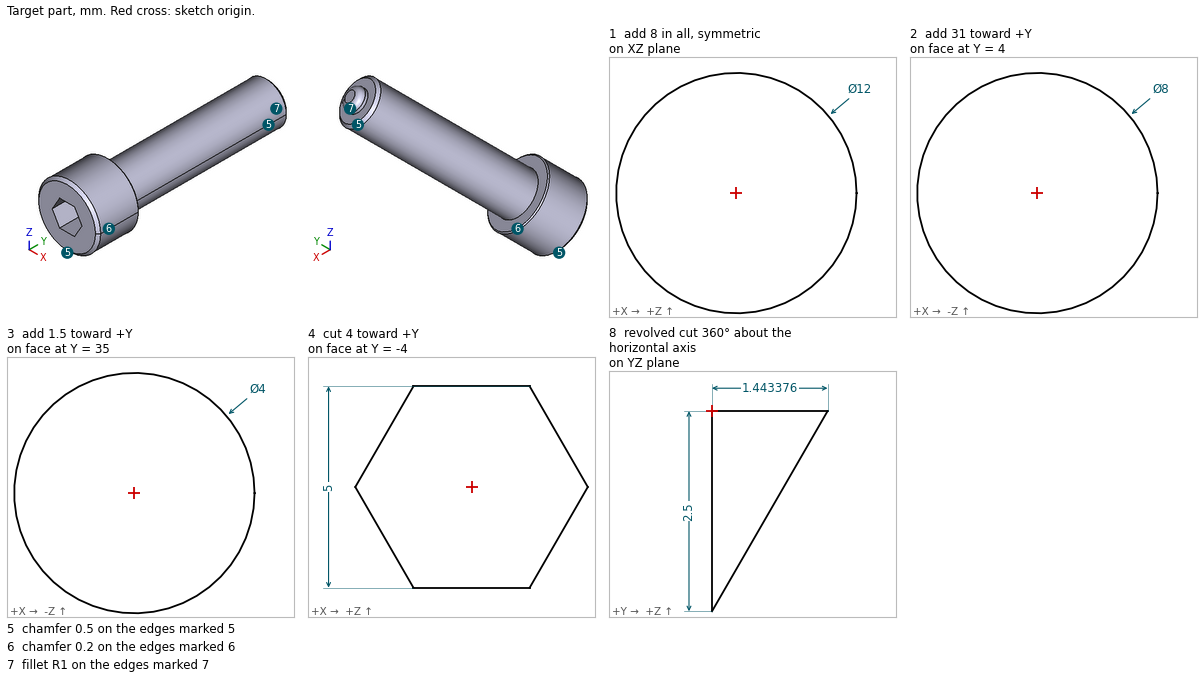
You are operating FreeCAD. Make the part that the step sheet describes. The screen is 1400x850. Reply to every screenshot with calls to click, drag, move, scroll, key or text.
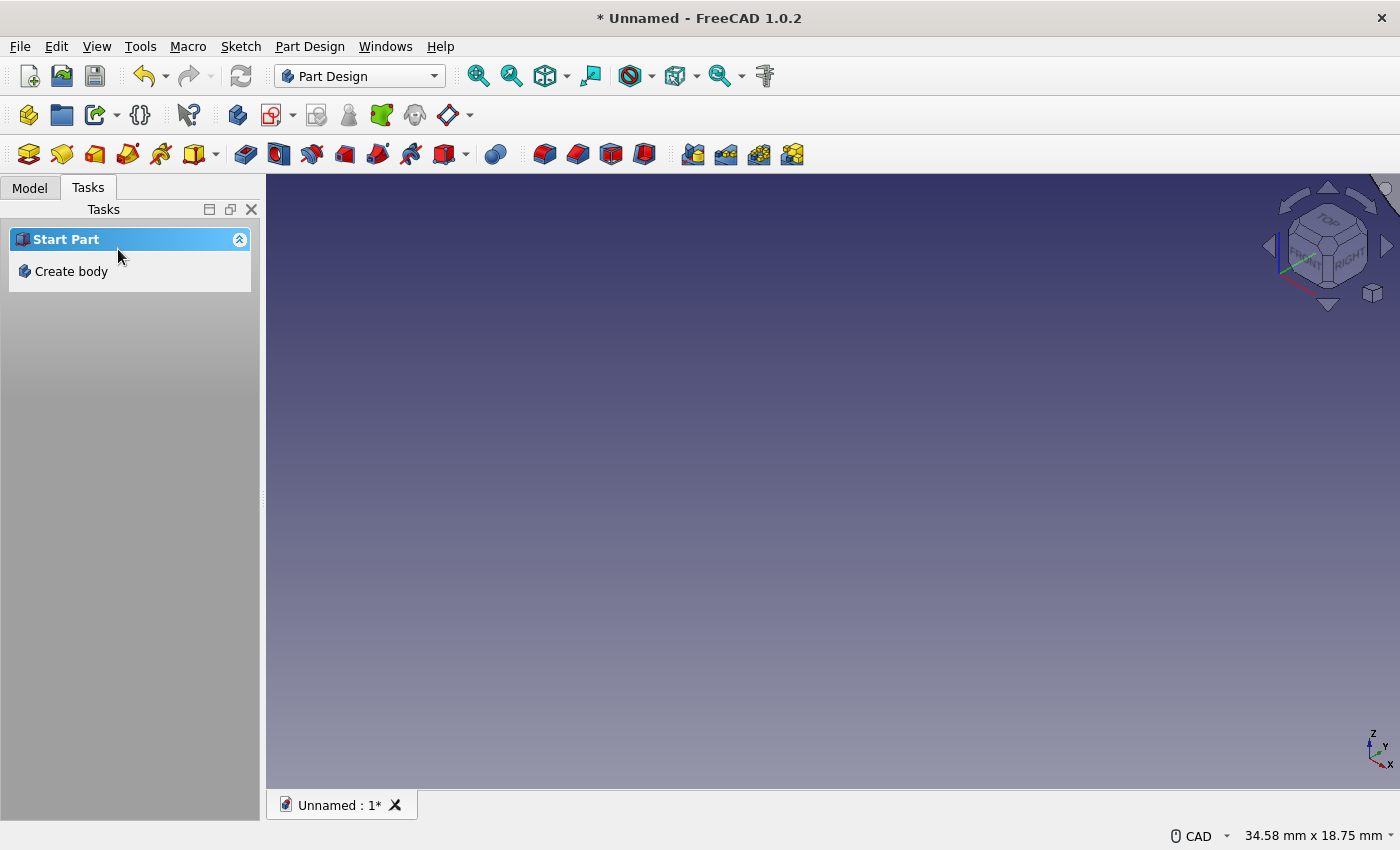
click(479, 76)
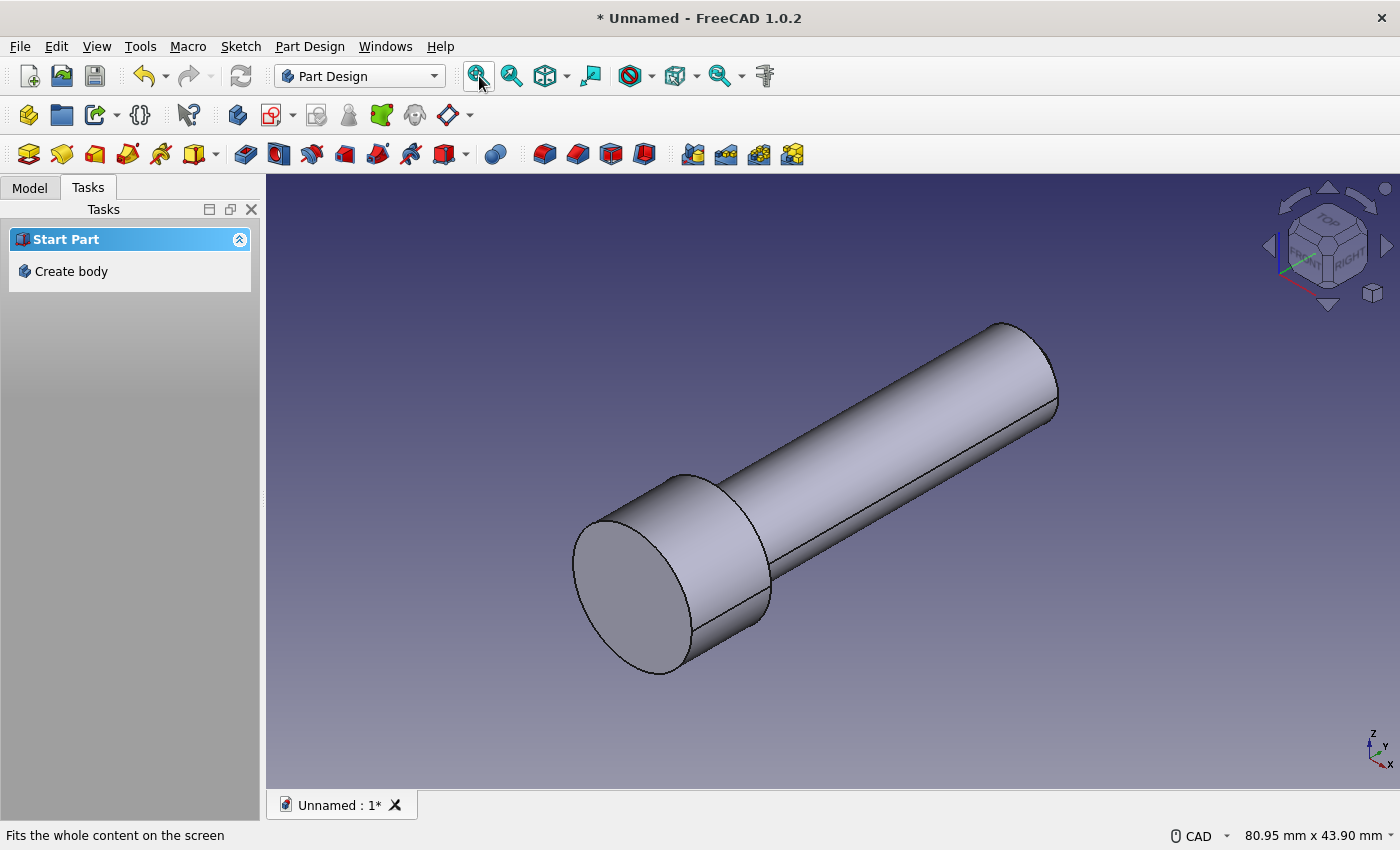
click(632, 596)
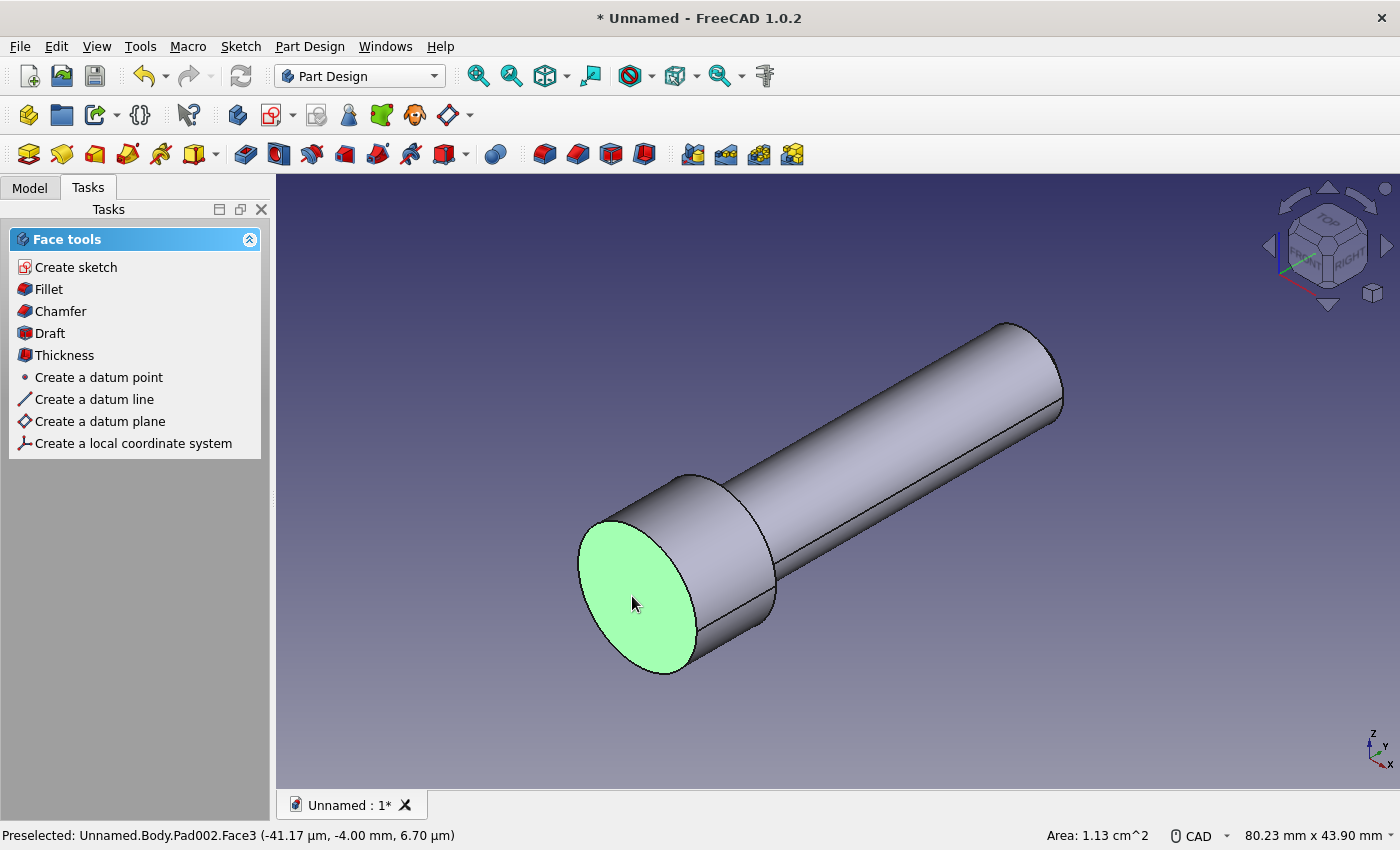
click(270, 116)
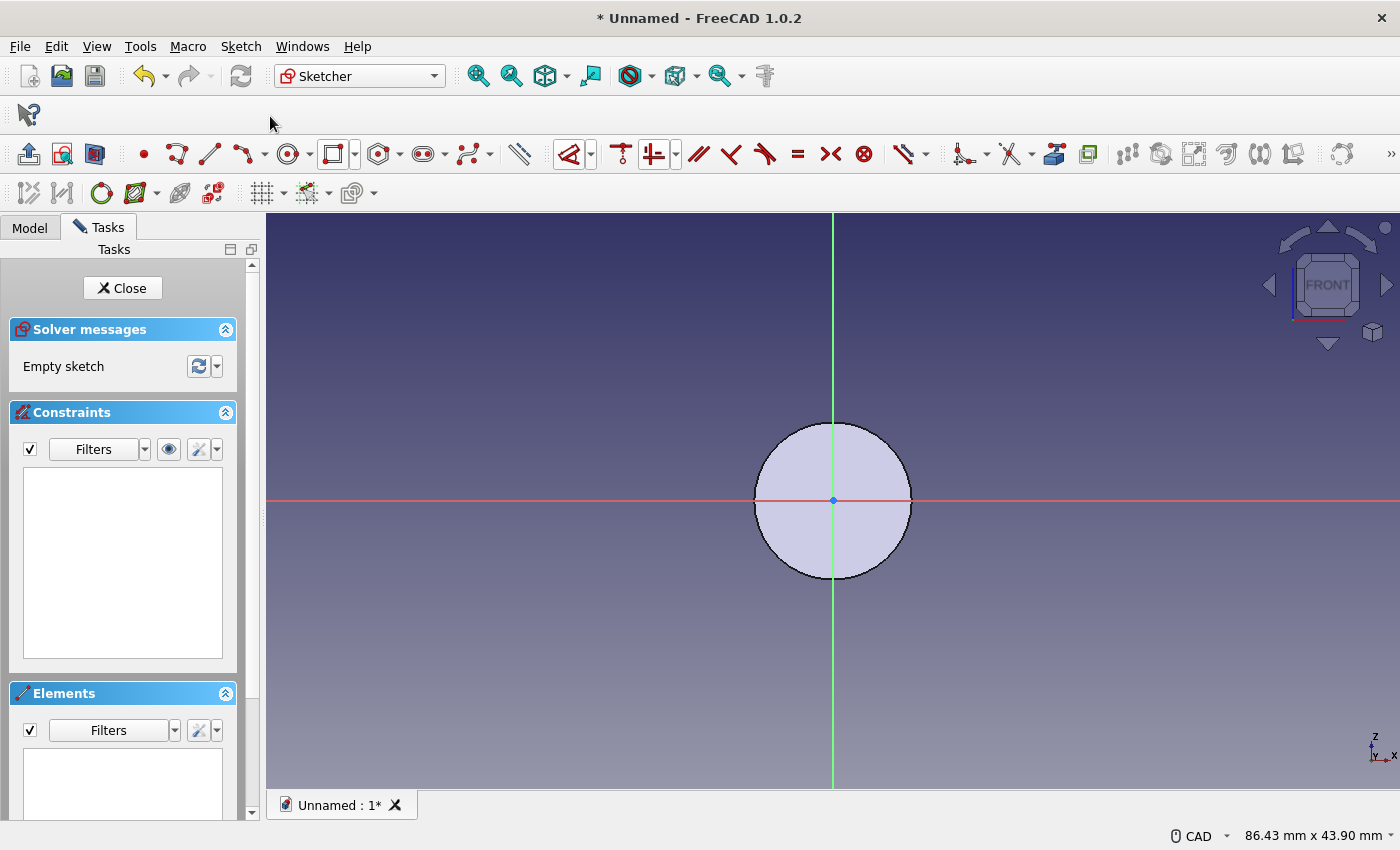
scroll(847, 501, up, 9)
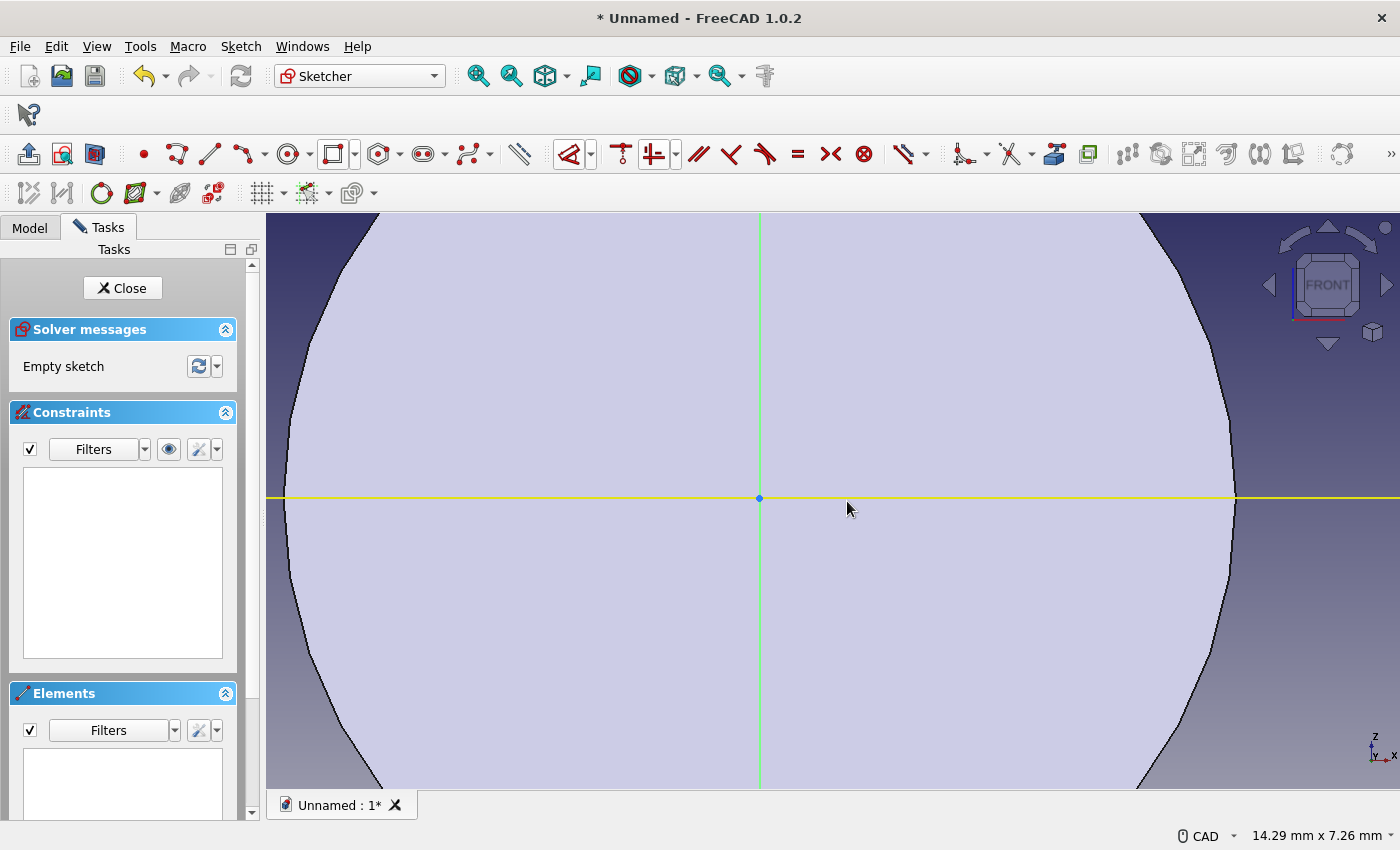
click(378, 154)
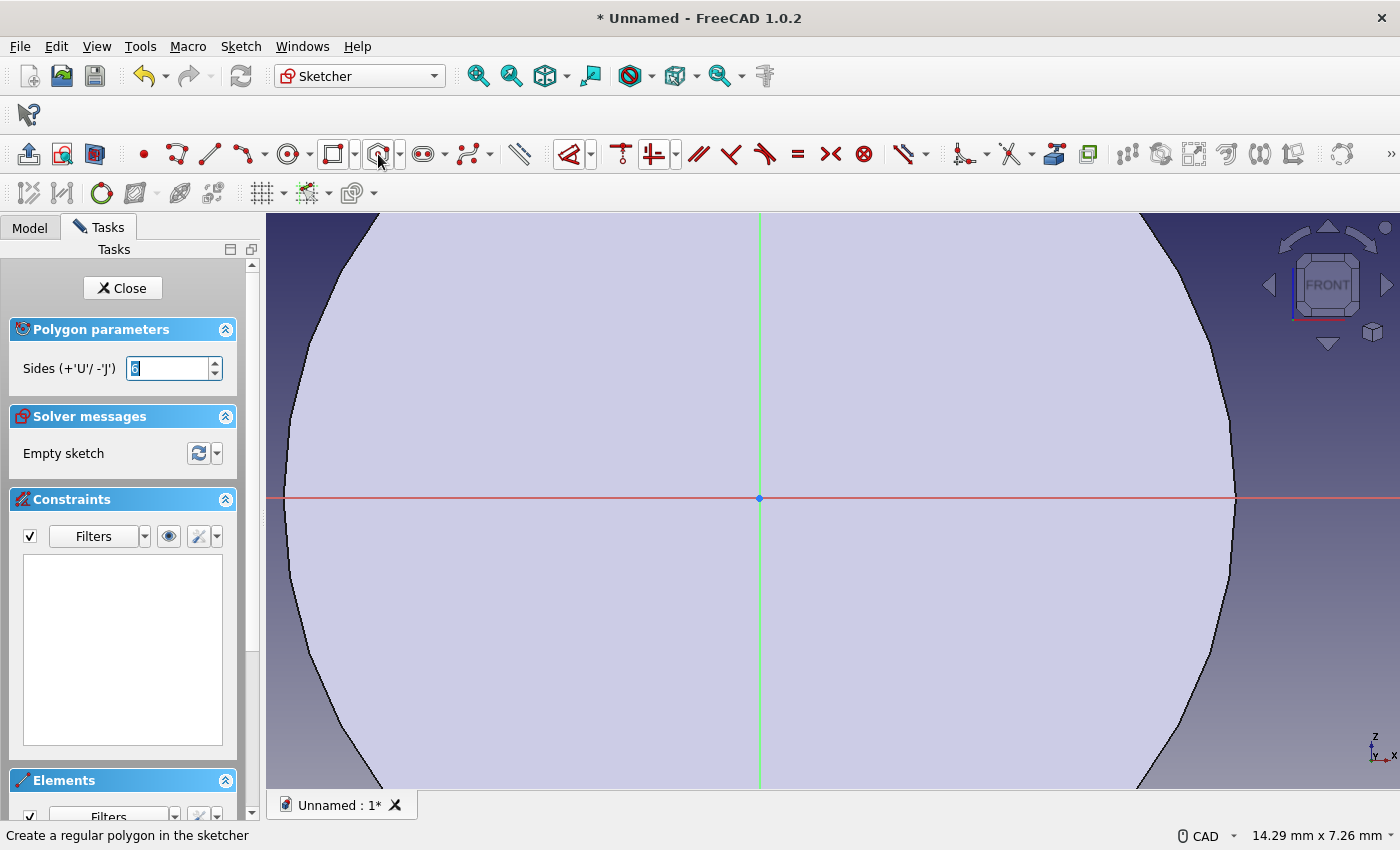
click(760, 498)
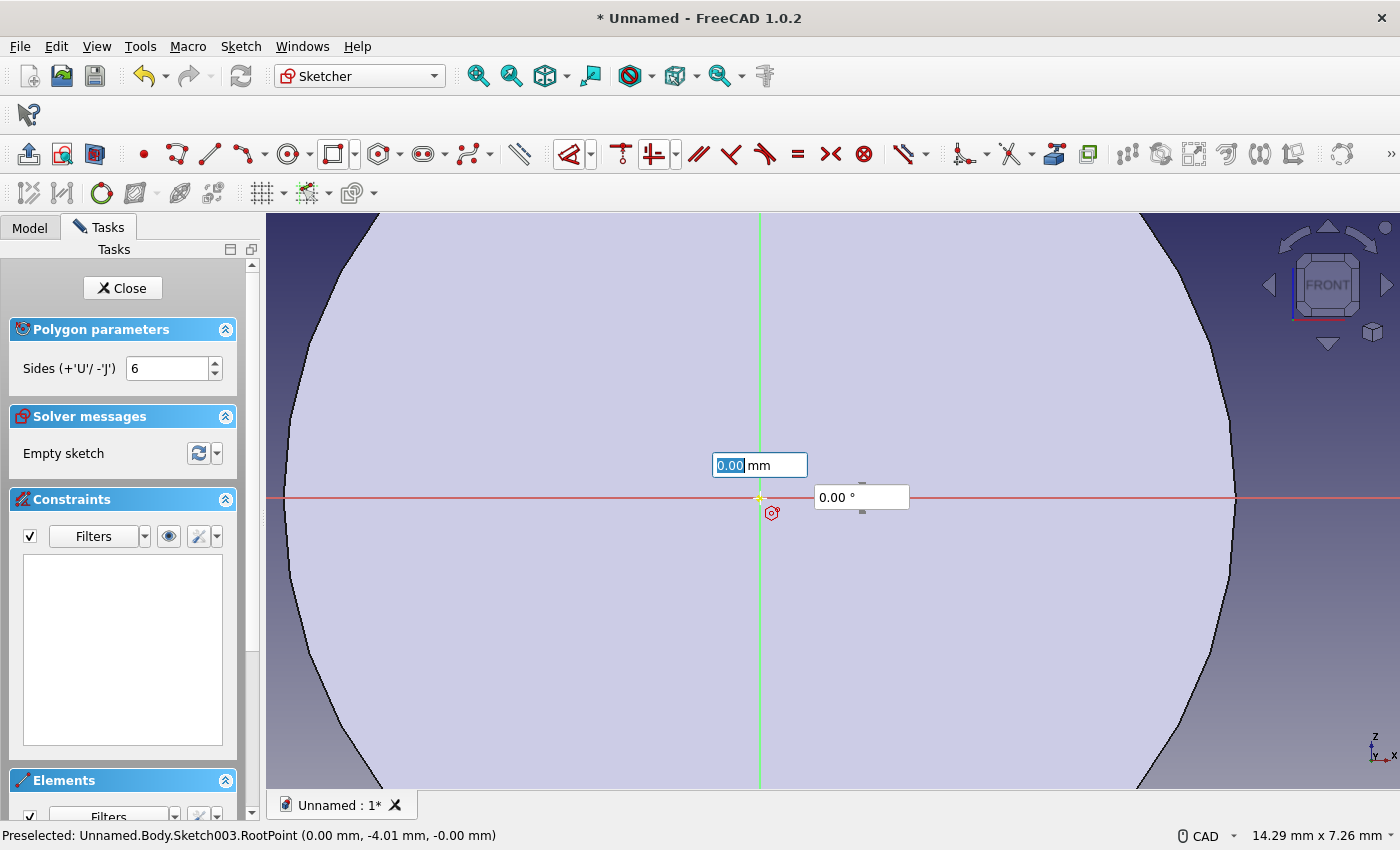
click(989, 498)
key(Escape)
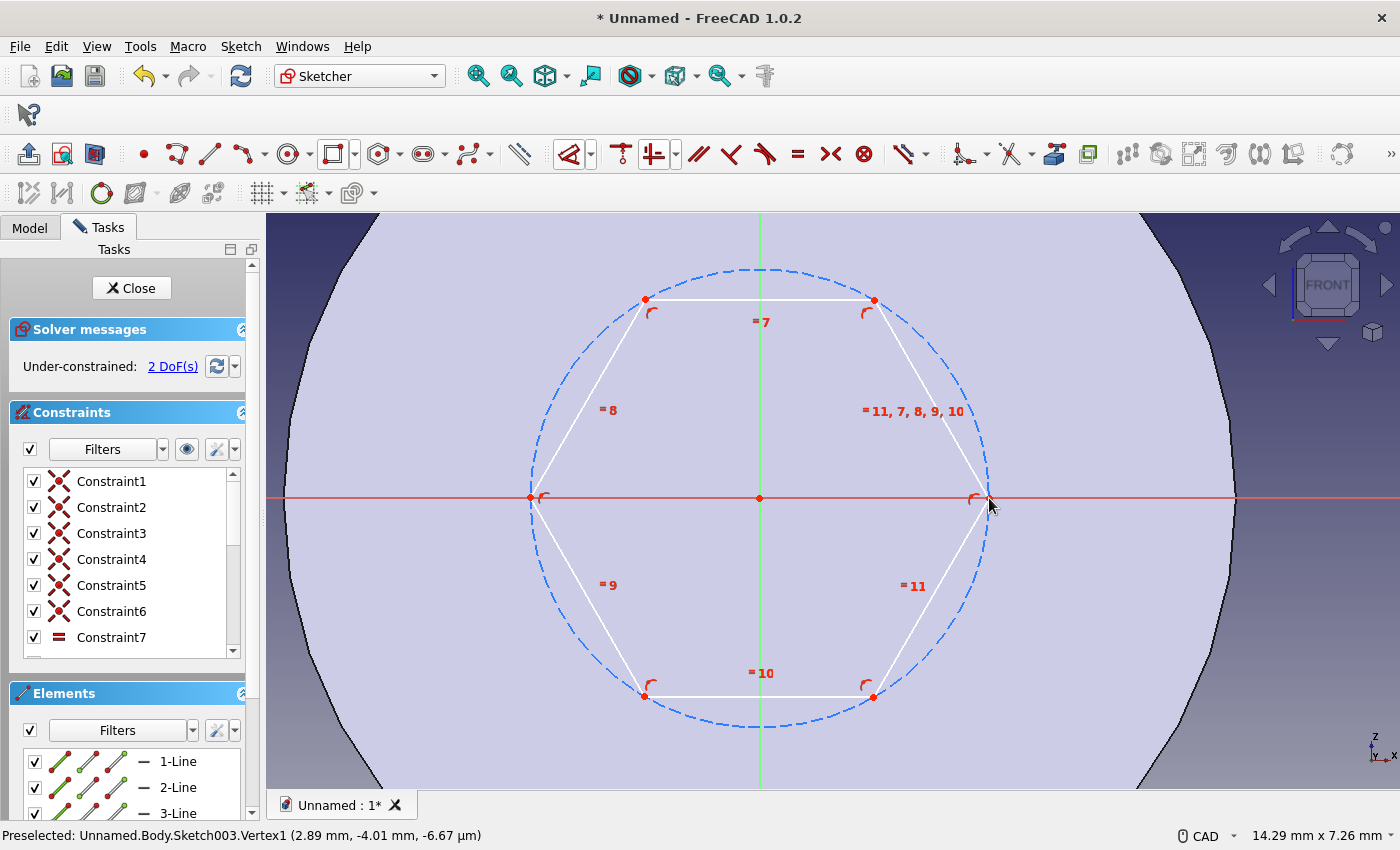
click(806, 300)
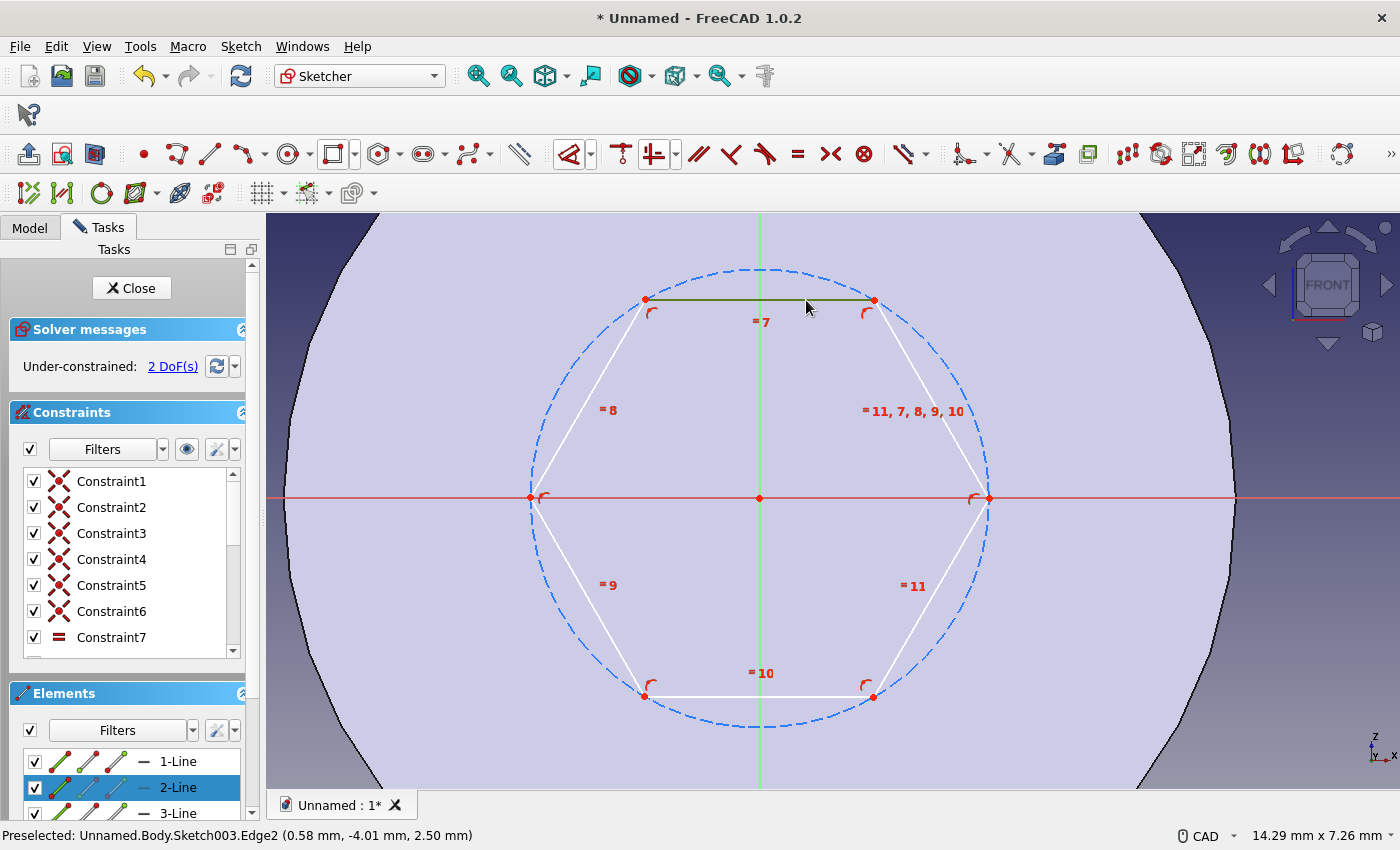
click(676, 154)